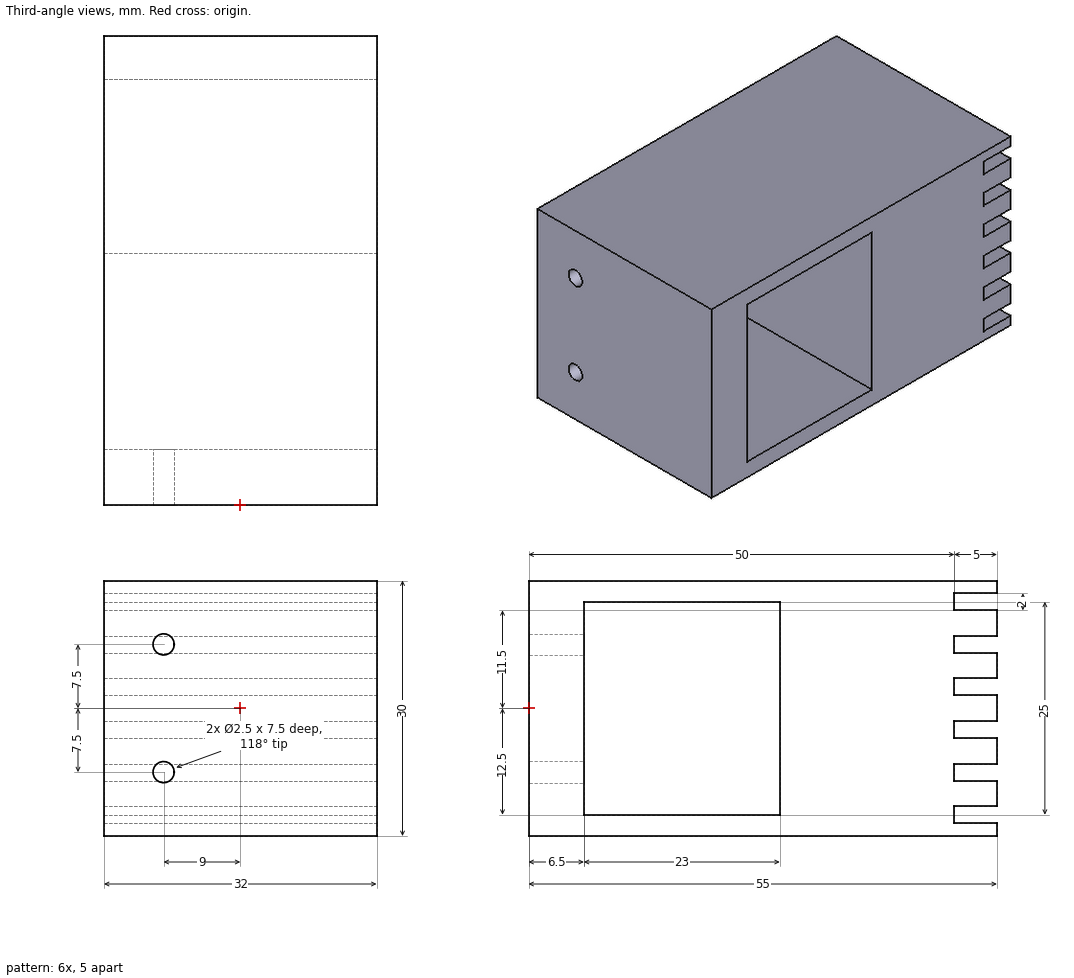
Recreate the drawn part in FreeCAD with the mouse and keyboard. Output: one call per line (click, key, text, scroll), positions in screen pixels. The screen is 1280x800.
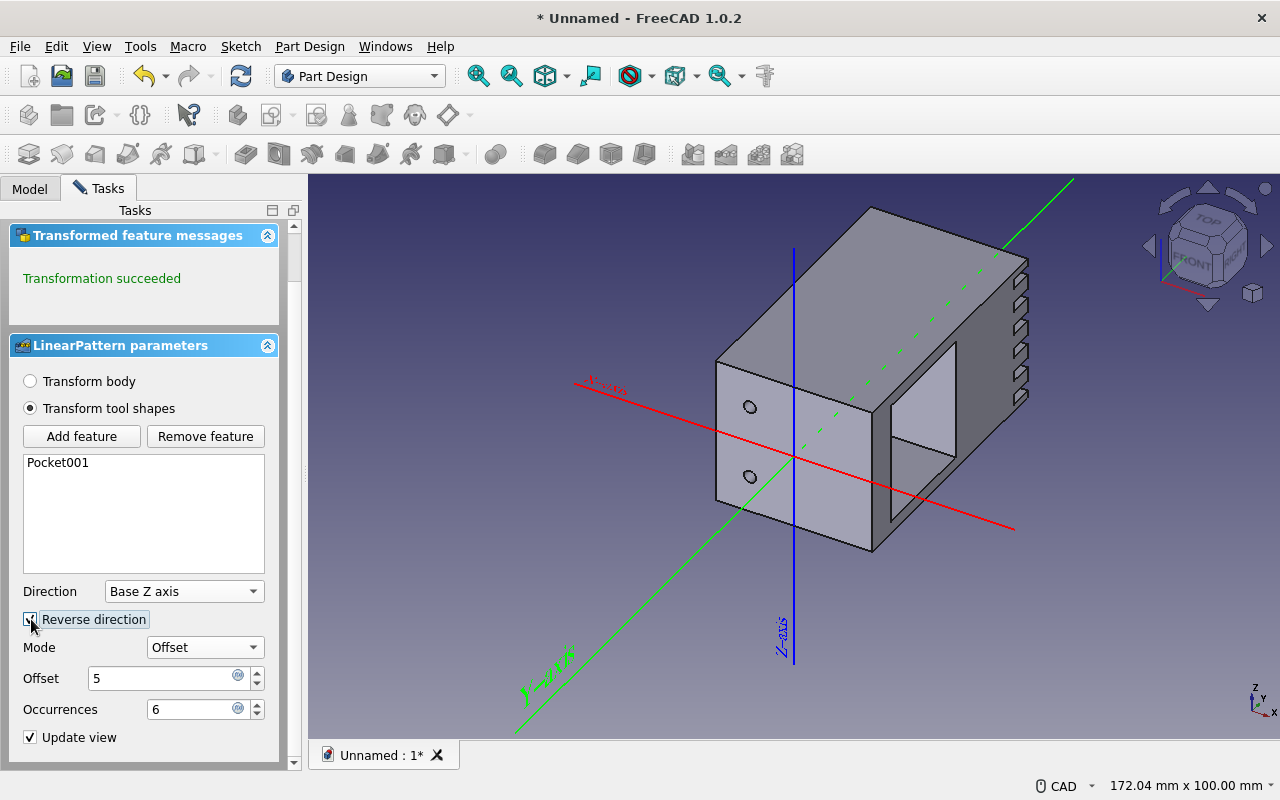
scroll(294, 495, up, 2)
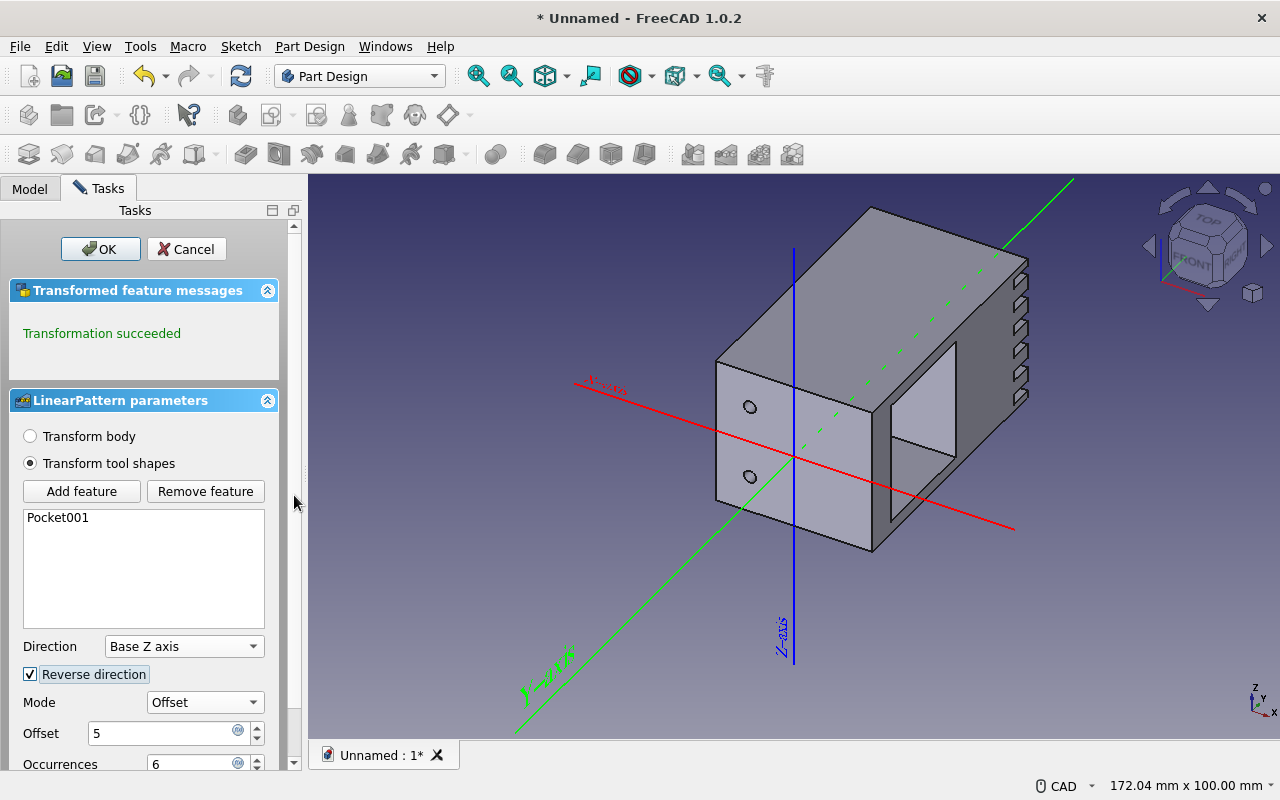
click(101, 249)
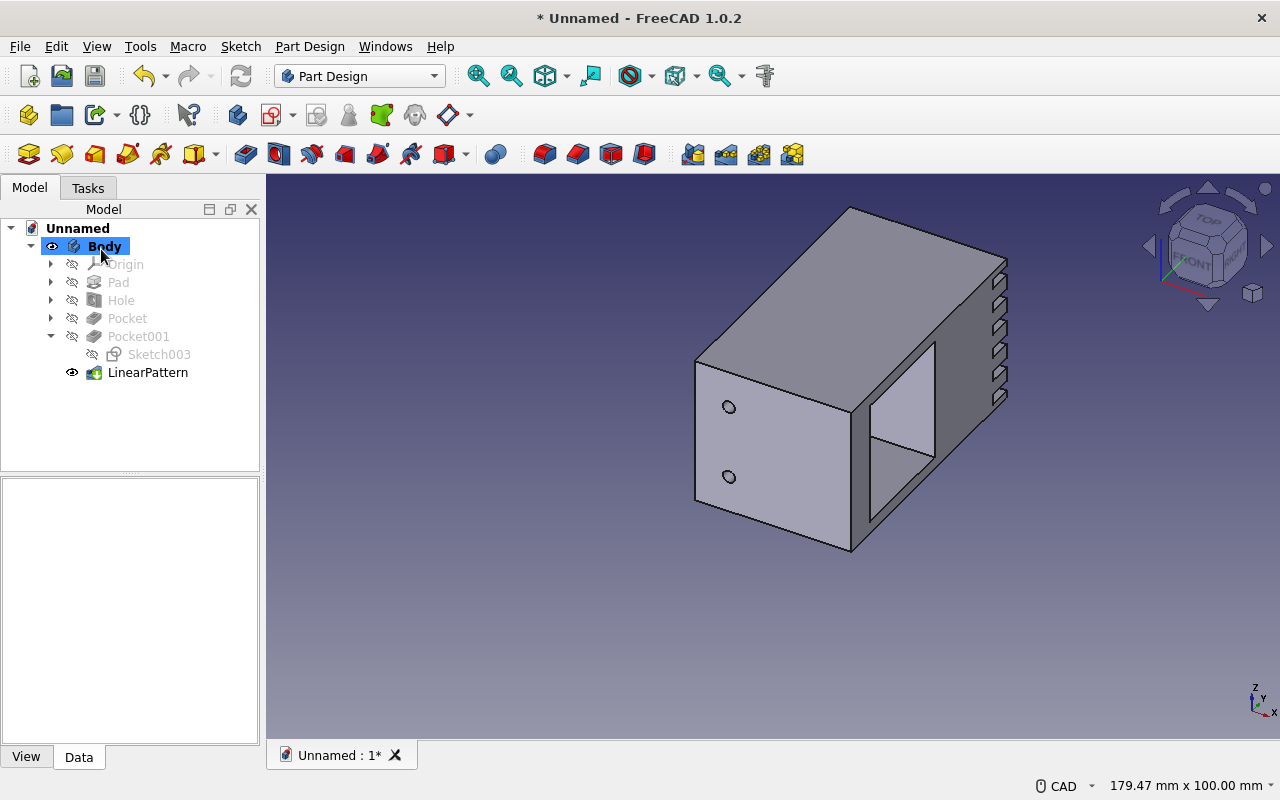
key(0)